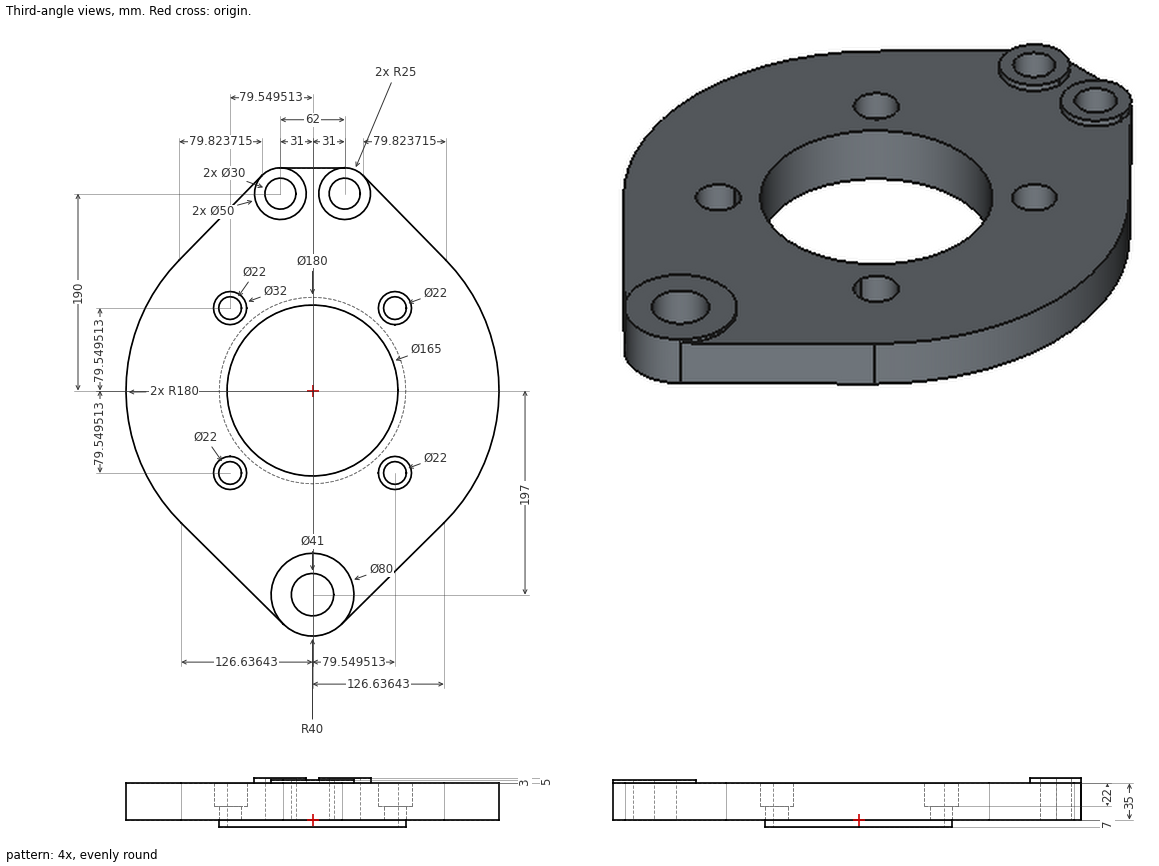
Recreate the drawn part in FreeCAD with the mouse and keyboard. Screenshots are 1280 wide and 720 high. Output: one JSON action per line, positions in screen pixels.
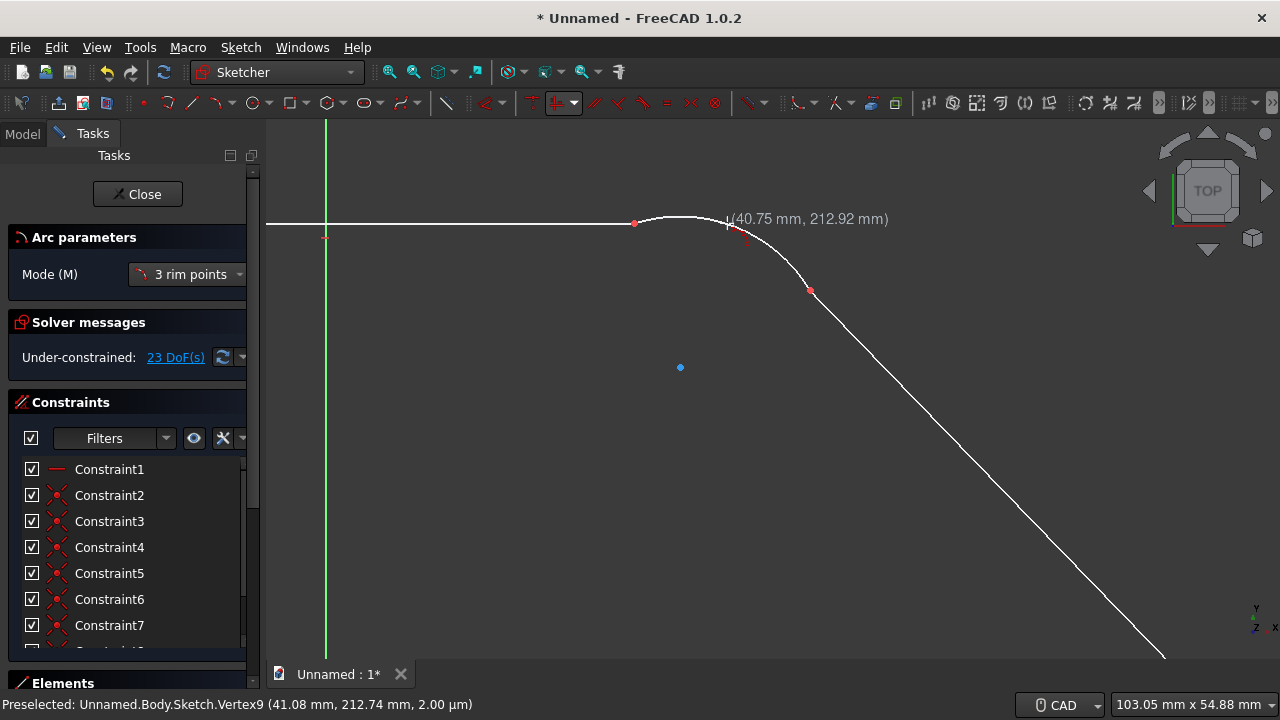
{"action": "scroll", "coordinate": [735, 225], "scroll_direction": "down", "scroll_amount": 13}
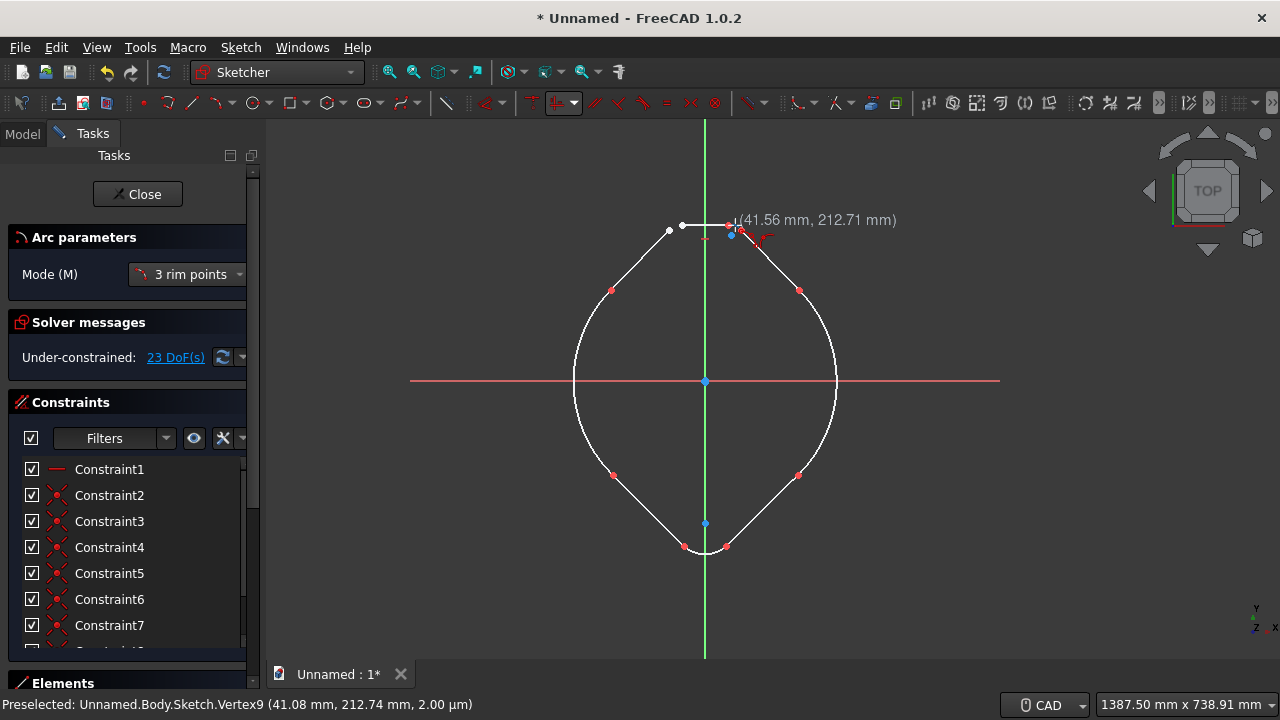
{"action": "left_click", "coordinate": [682, 225]}
{"action": "left_click", "coordinate": [669, 230]}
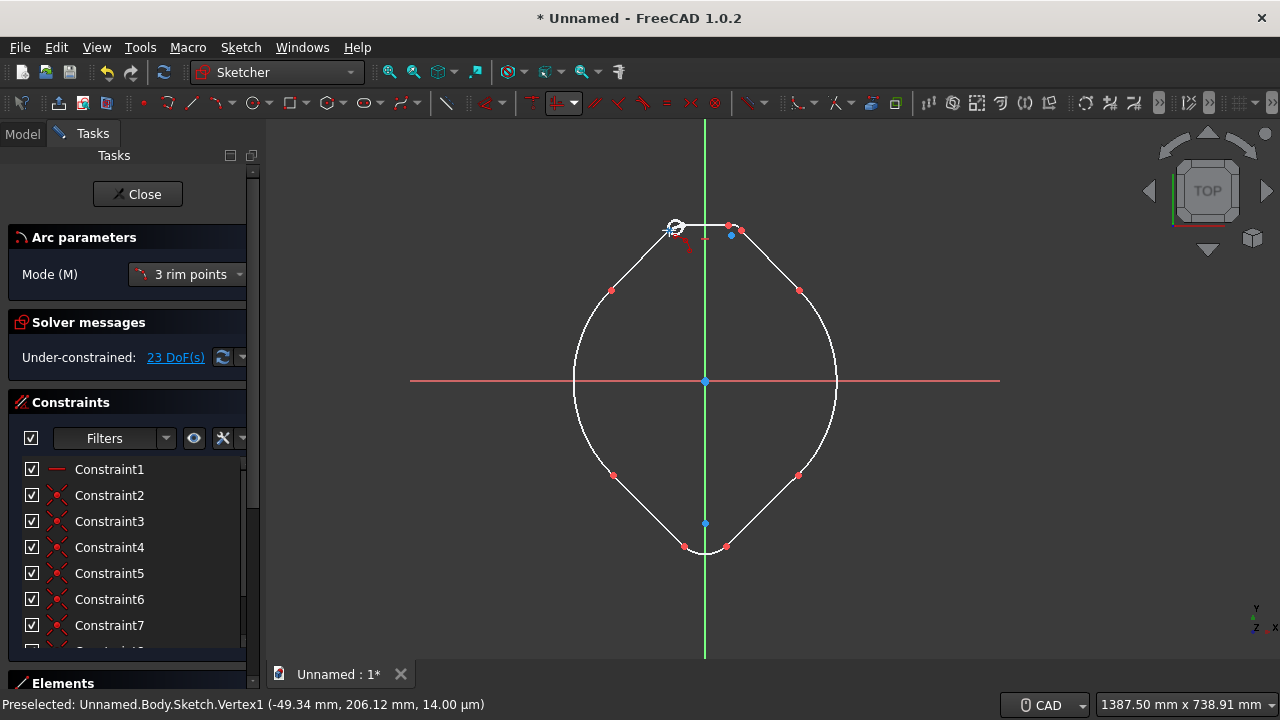
{"action": "scroll", "coordinate": [675, 225], "scroll_direction": "up", "scroll_amount": 13}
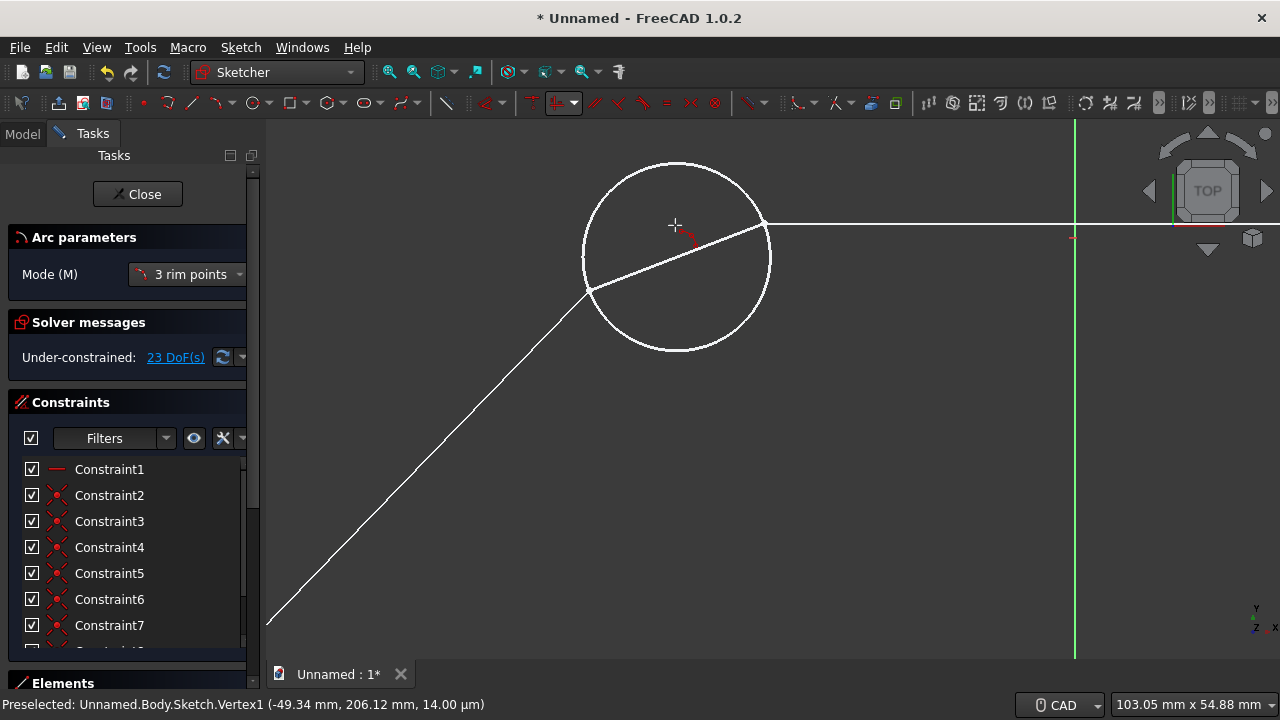
{"action": "left_click", "coordinate": [674, 223]}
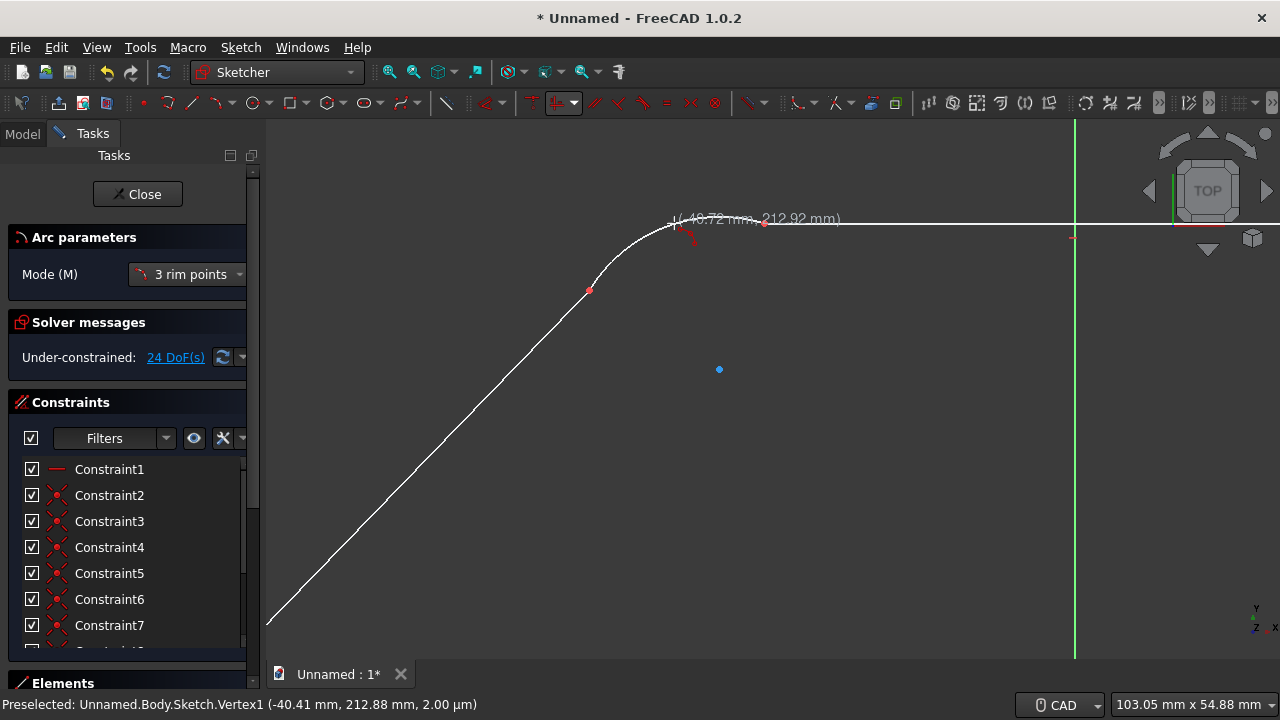
{"action": "key", "text": "g c"}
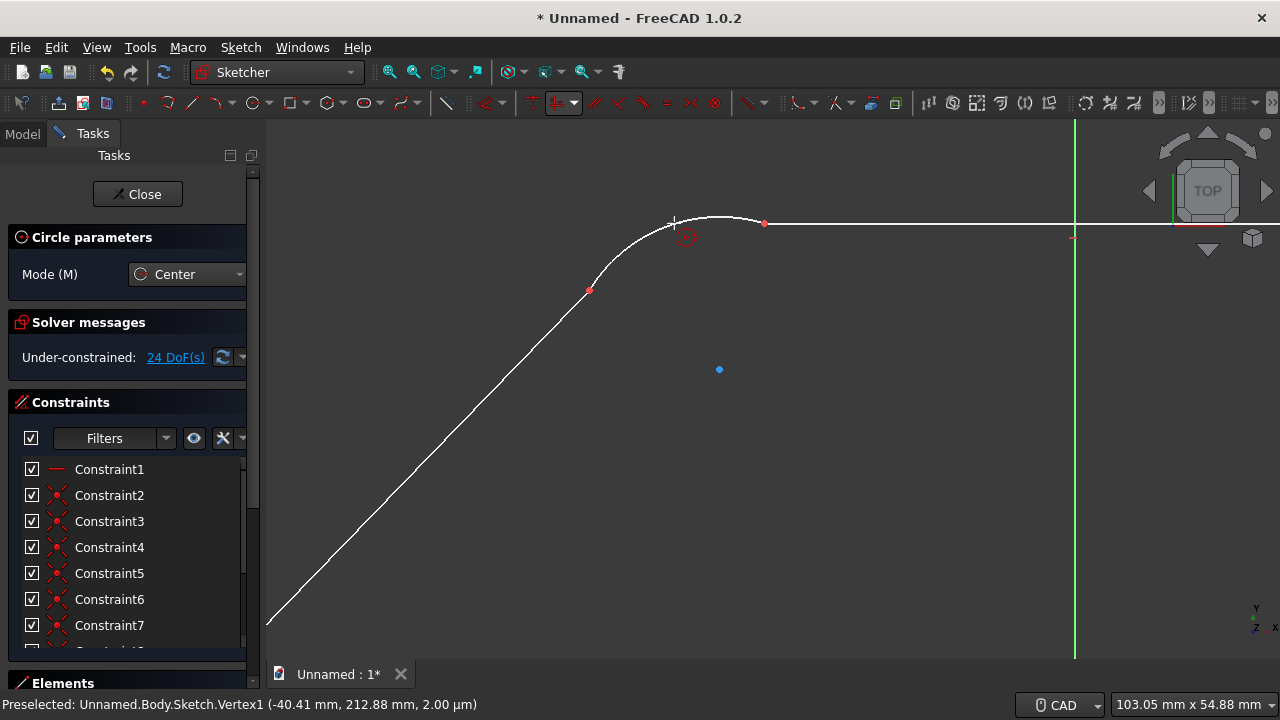
{"action": "scroll", "coordinate": [675, 225], "scroll_direction": "down", "scroll_amount": 13}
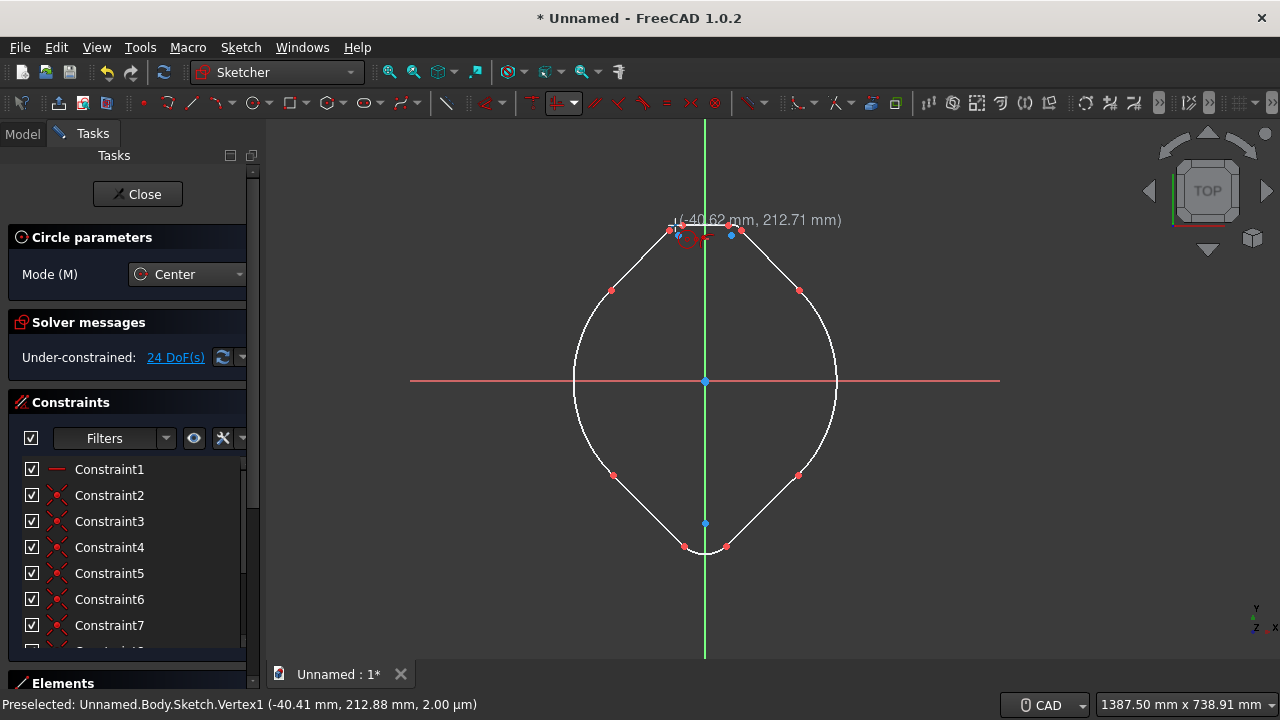
{"action": "scroll", "coordinate": [705, 525], "scroll_direction": "up", "scroll_amount": 3}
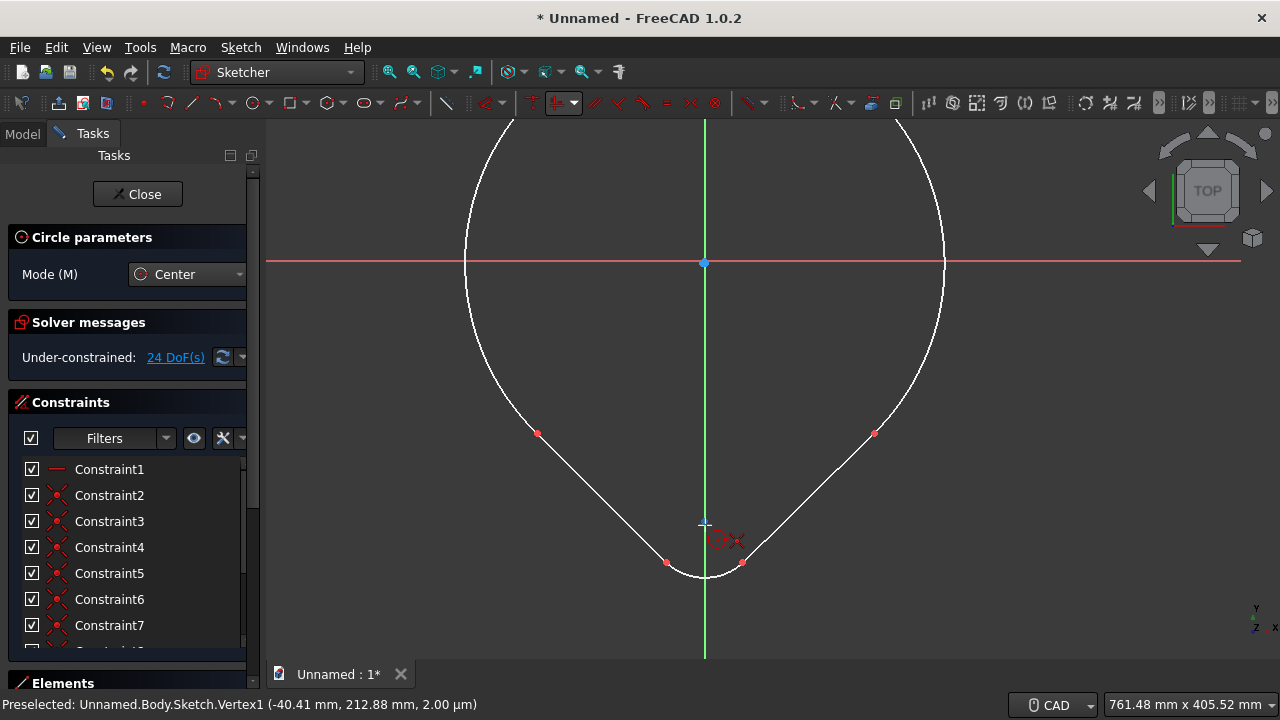
{"action": "left_click", "coordinate": [705, 524]}
{"action": "left_click", "coordinate": [724, 504]}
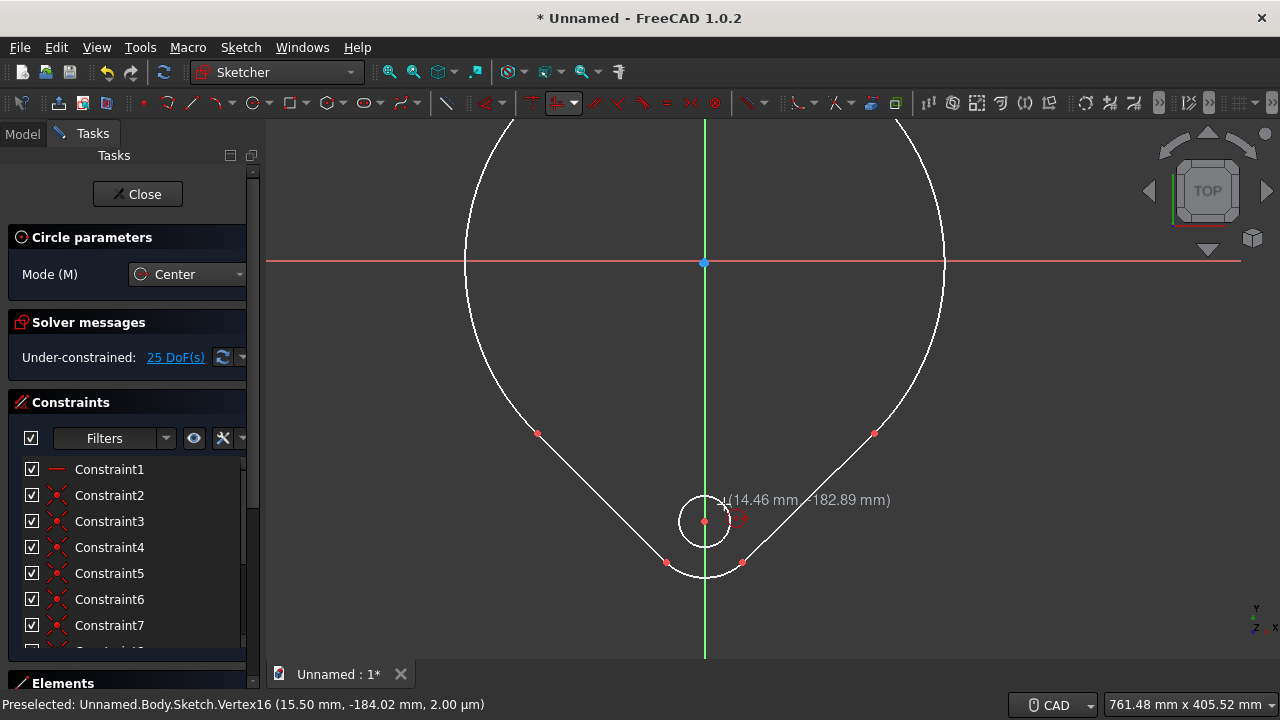
{"action": "scroll", "coordinate": [704, 526], "scroll_direction": "down", "scroll_amount": 3}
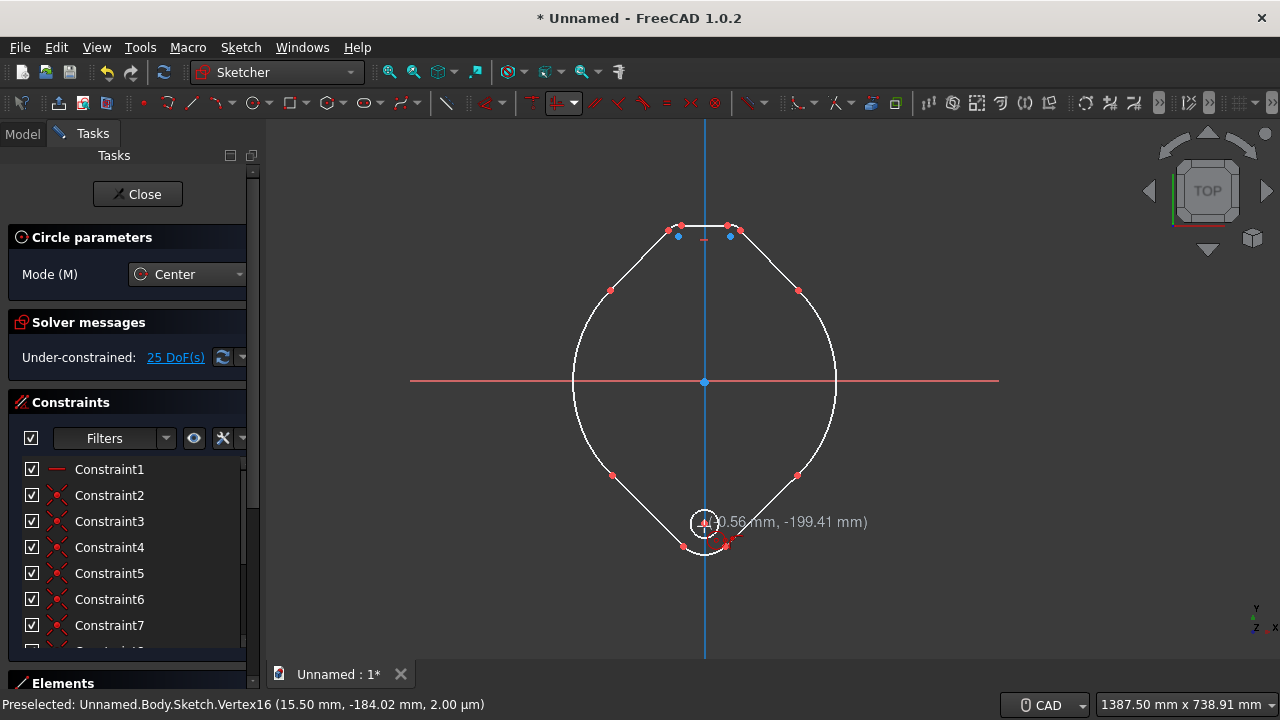
{"action": "scroll", "coordinate": [682, 242], "scroll_direction": "up", "scroll_amount": 4}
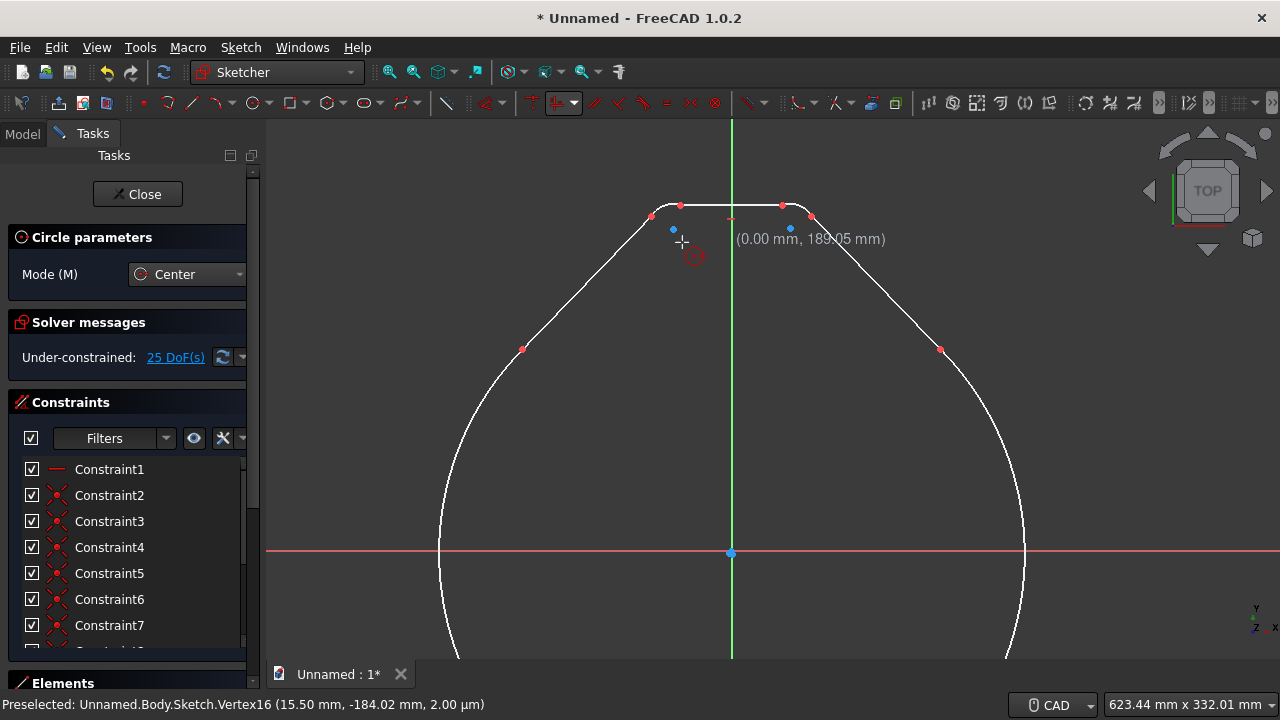
{"action": "left_click", "coordinate": [681, 242]}
{"action": "left_click", "coordinate": [699, 225]}